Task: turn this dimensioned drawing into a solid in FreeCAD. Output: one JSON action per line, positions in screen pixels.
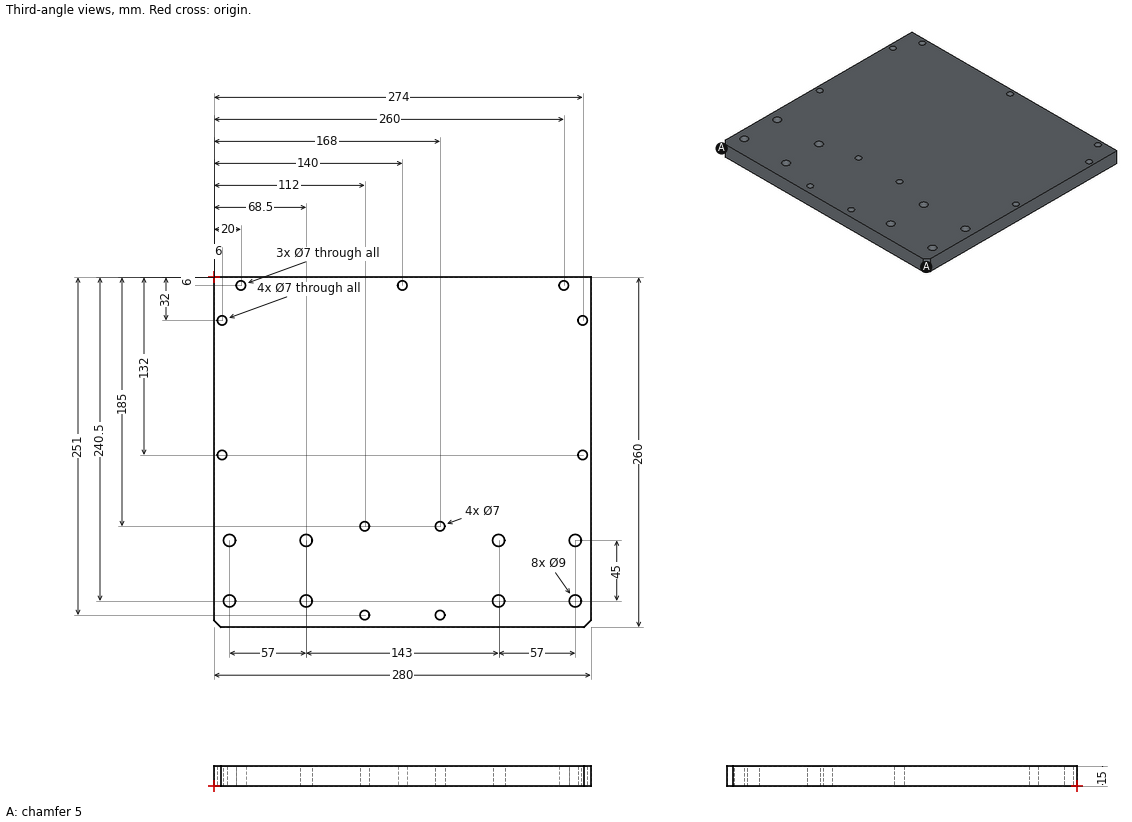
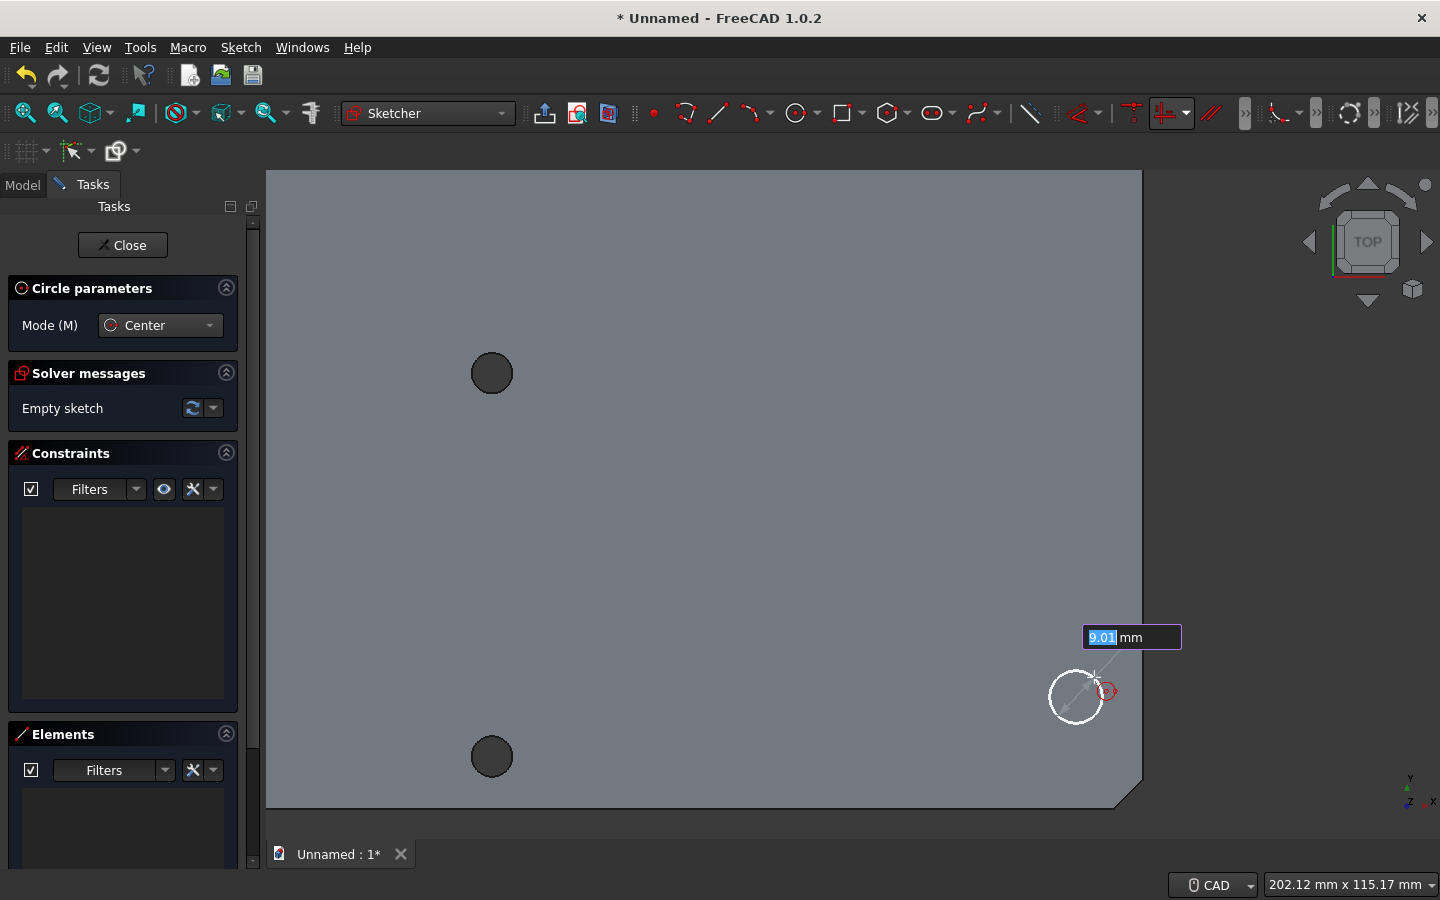
{"action": "type", "text": "9"}
{"action": "key", "text": "Return"}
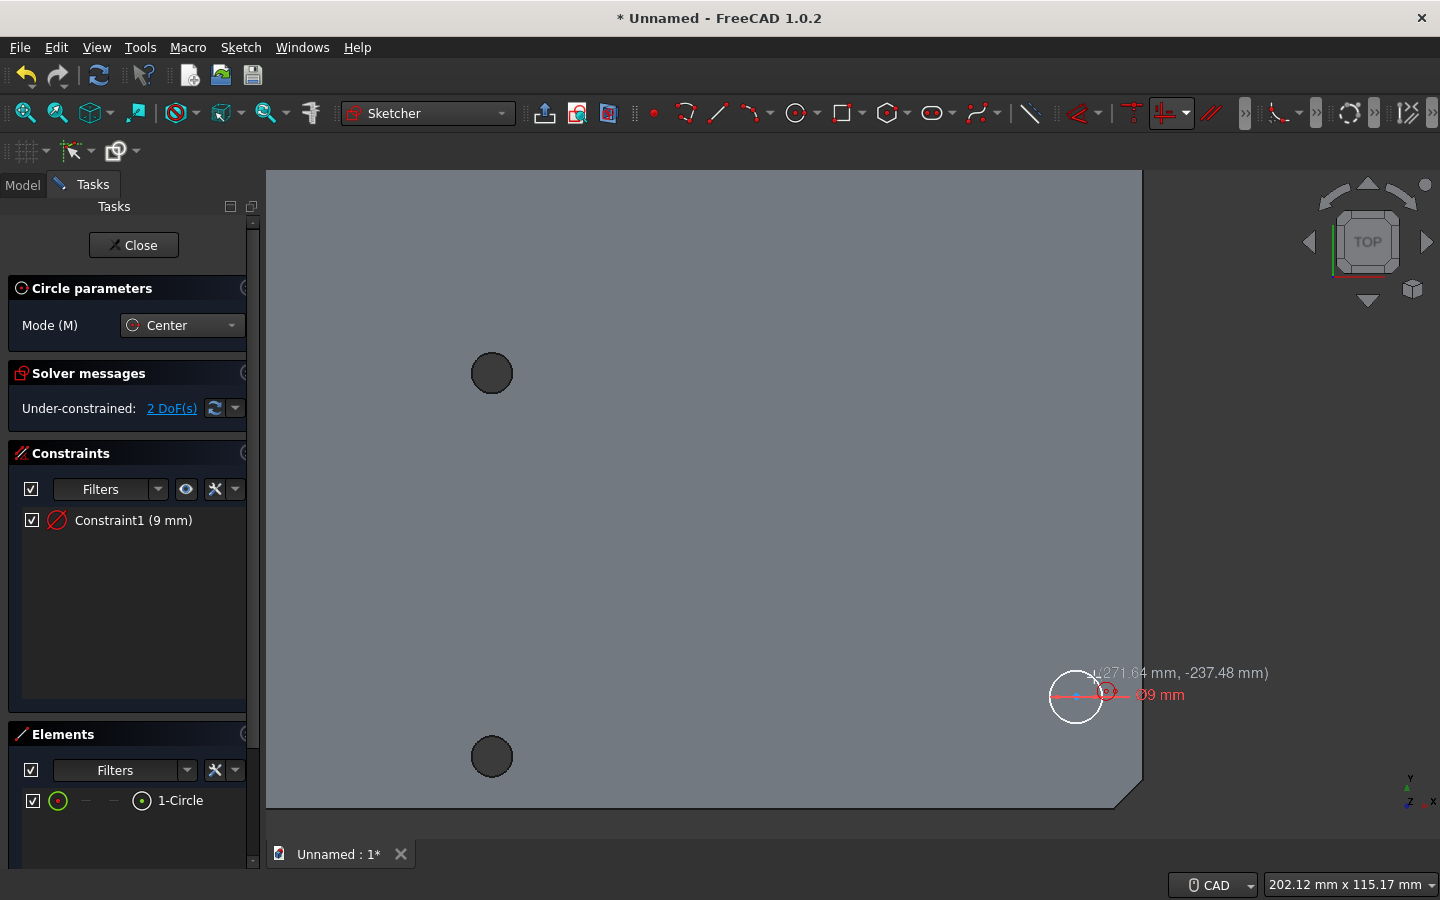
{"action": "left_click", "coordinate": [1076, 434]}
{"action": "mouse_move", "coordinate": [1094, 416]}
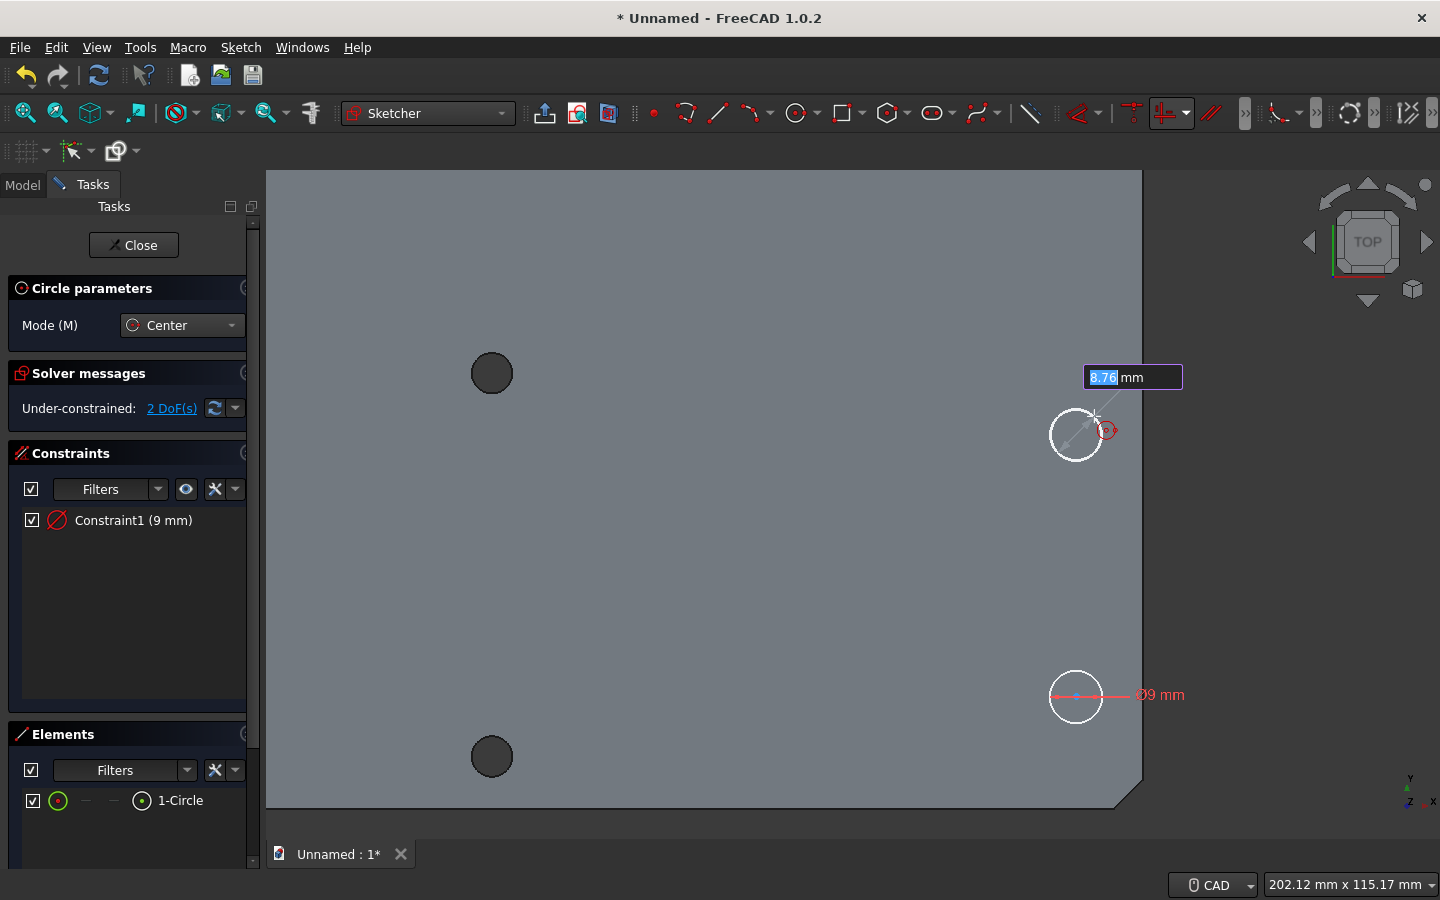
{"action": "type", "text": "9"}
{"action": "key", "text": "Return"}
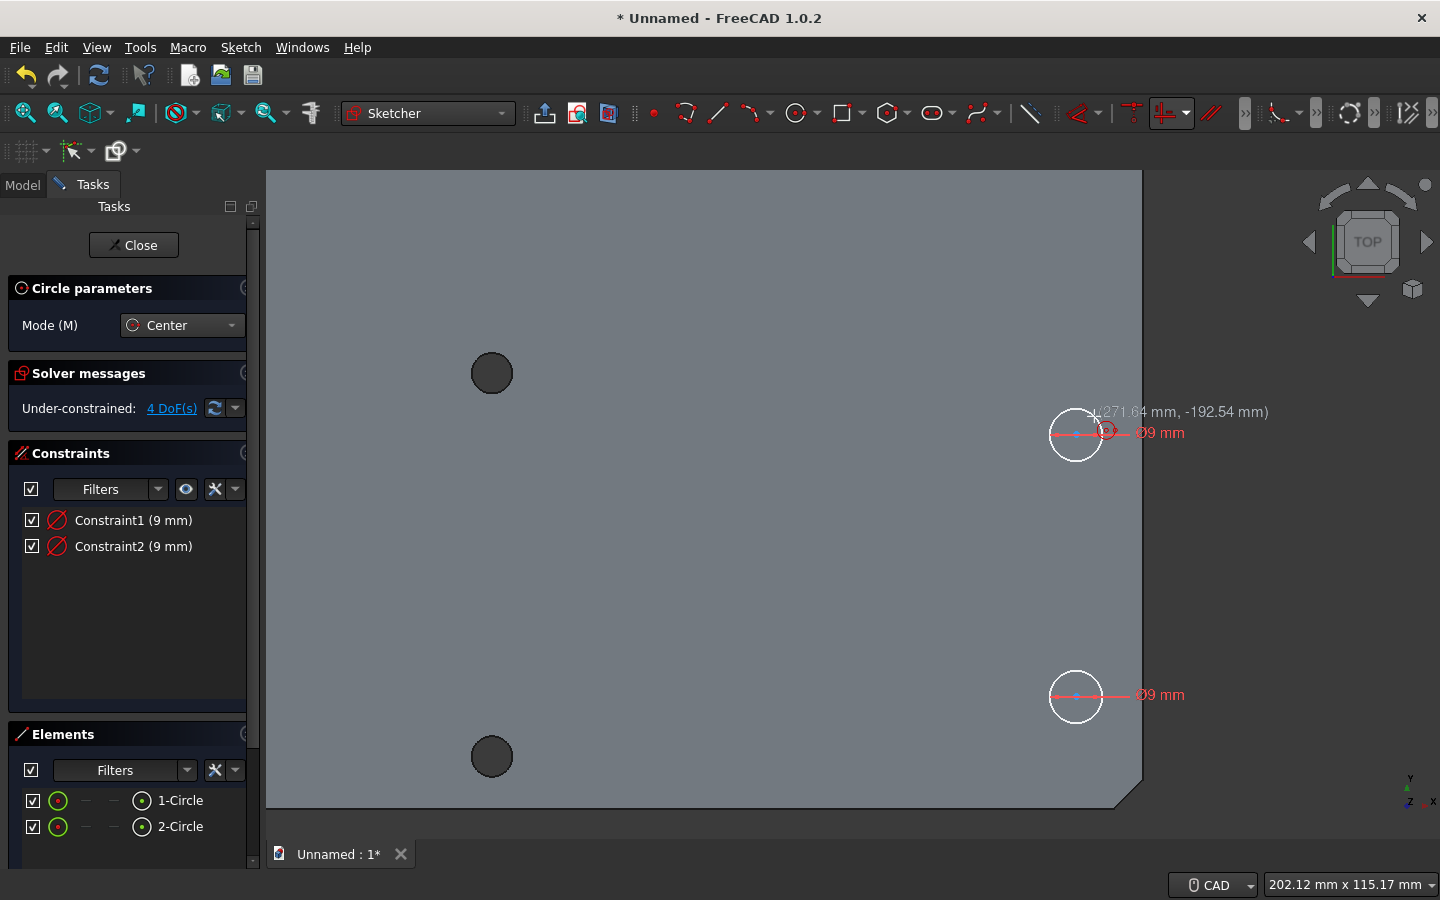
{"action": "left_click", "coordinate": [745, 434]}
{"action": "mouse_move", "coordinate": [763, 416]}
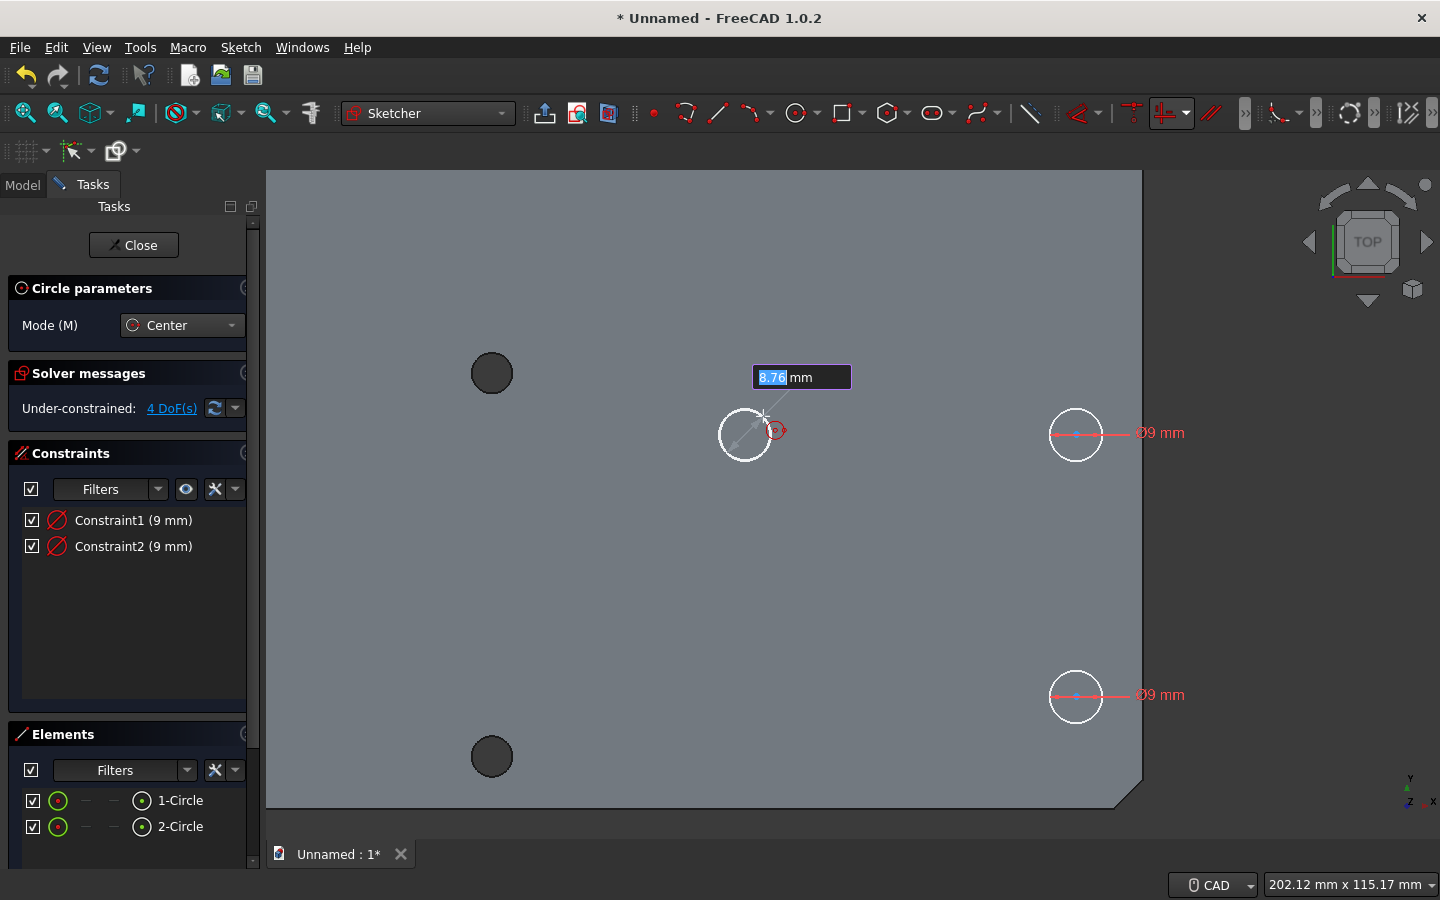
{"action": "type", "text": "9"}
{"action": "key", "text": "Return"}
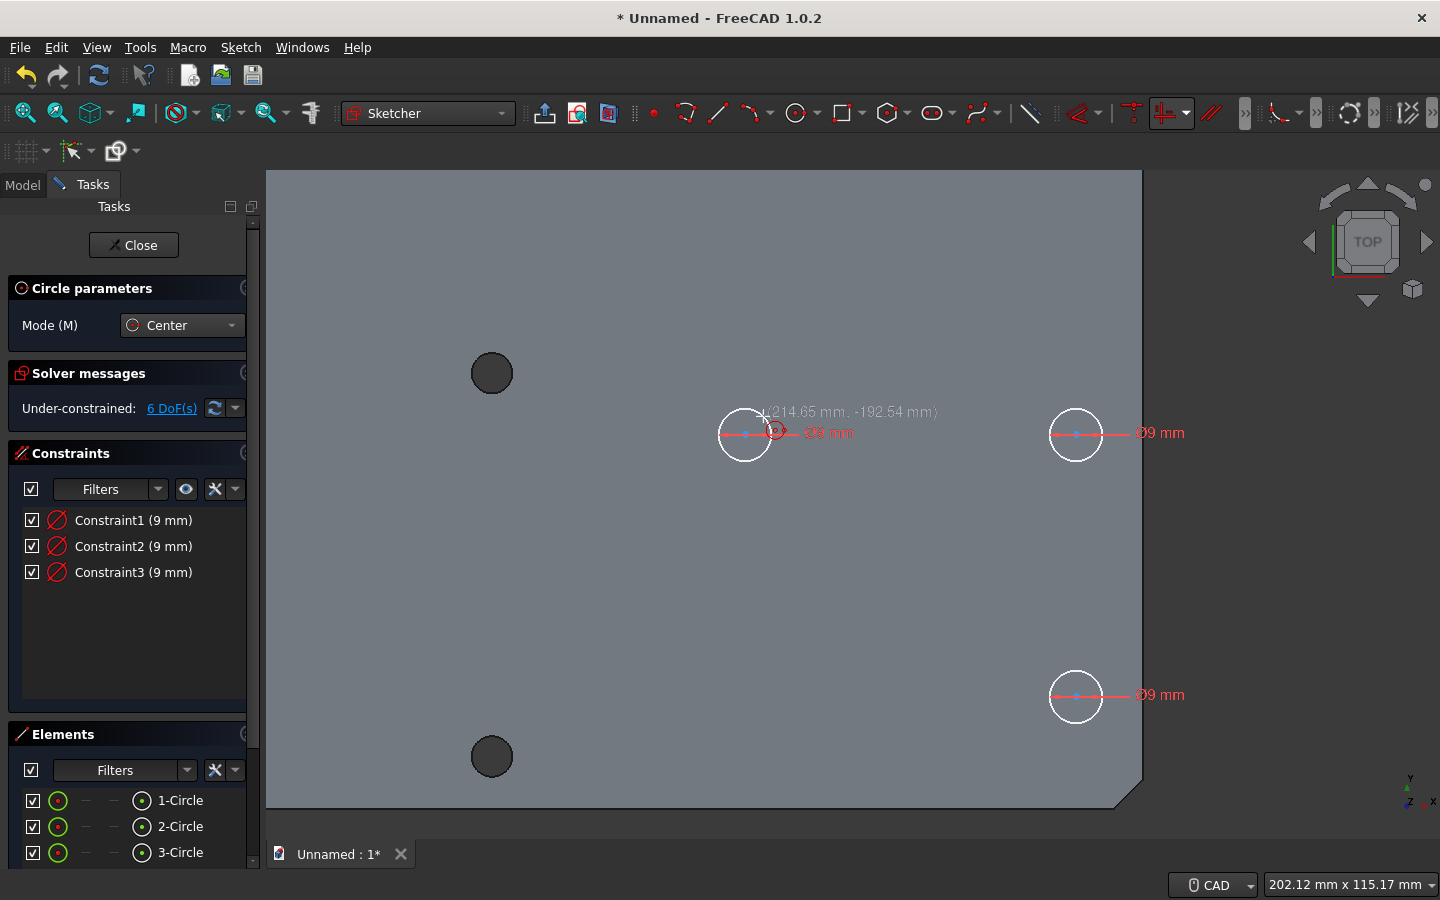
{"action": "left_click", "coordinate": [745, 696]}
{"action": "mouse_move", "coordinate": [763, 677]}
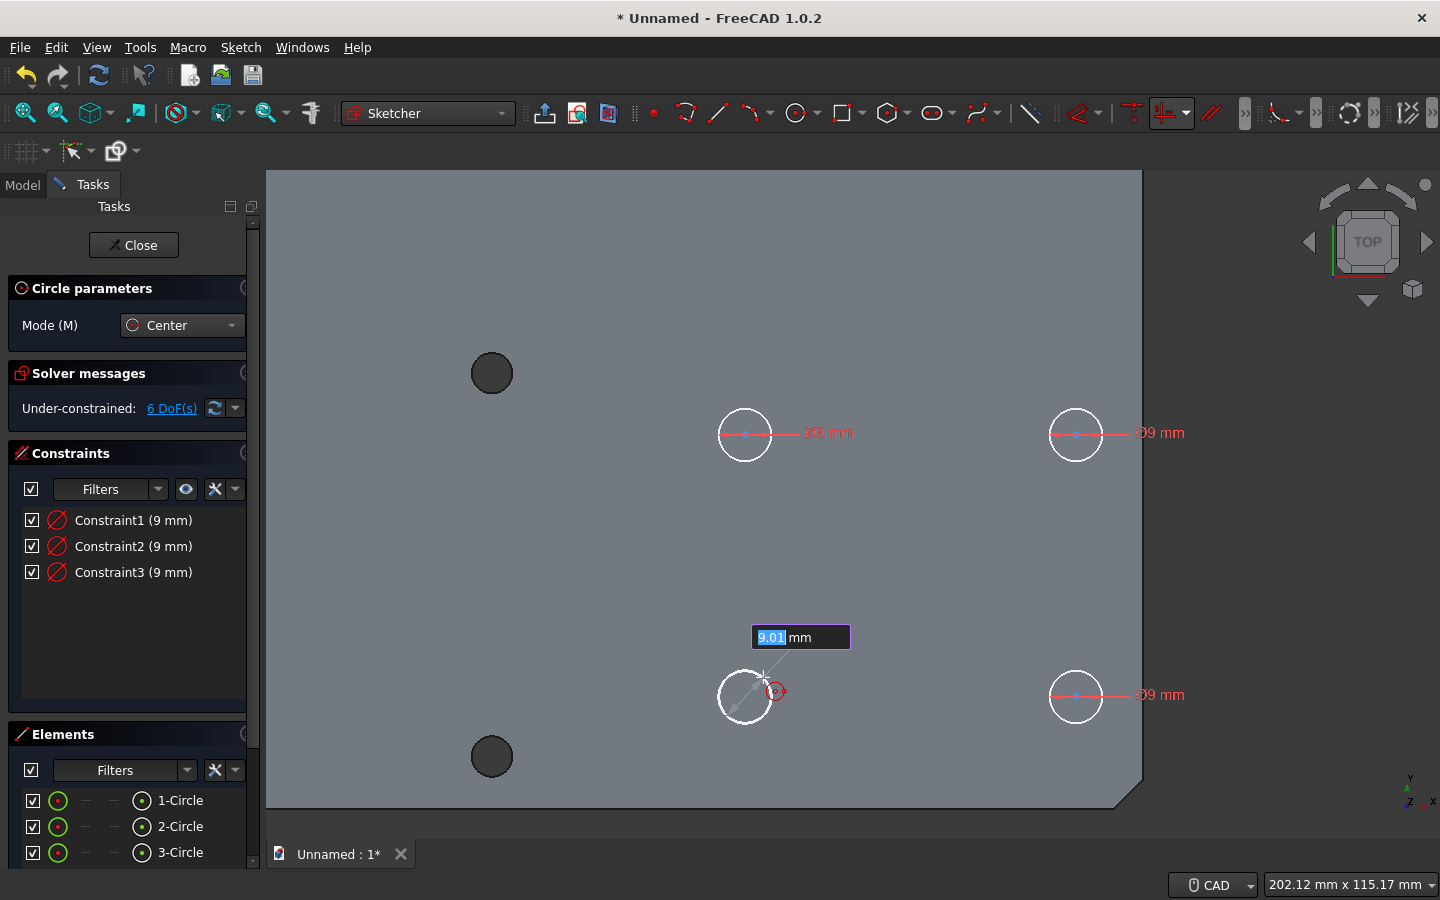
{"action": "type", "text": "9"}
{"action": "key", "text": "Return"}